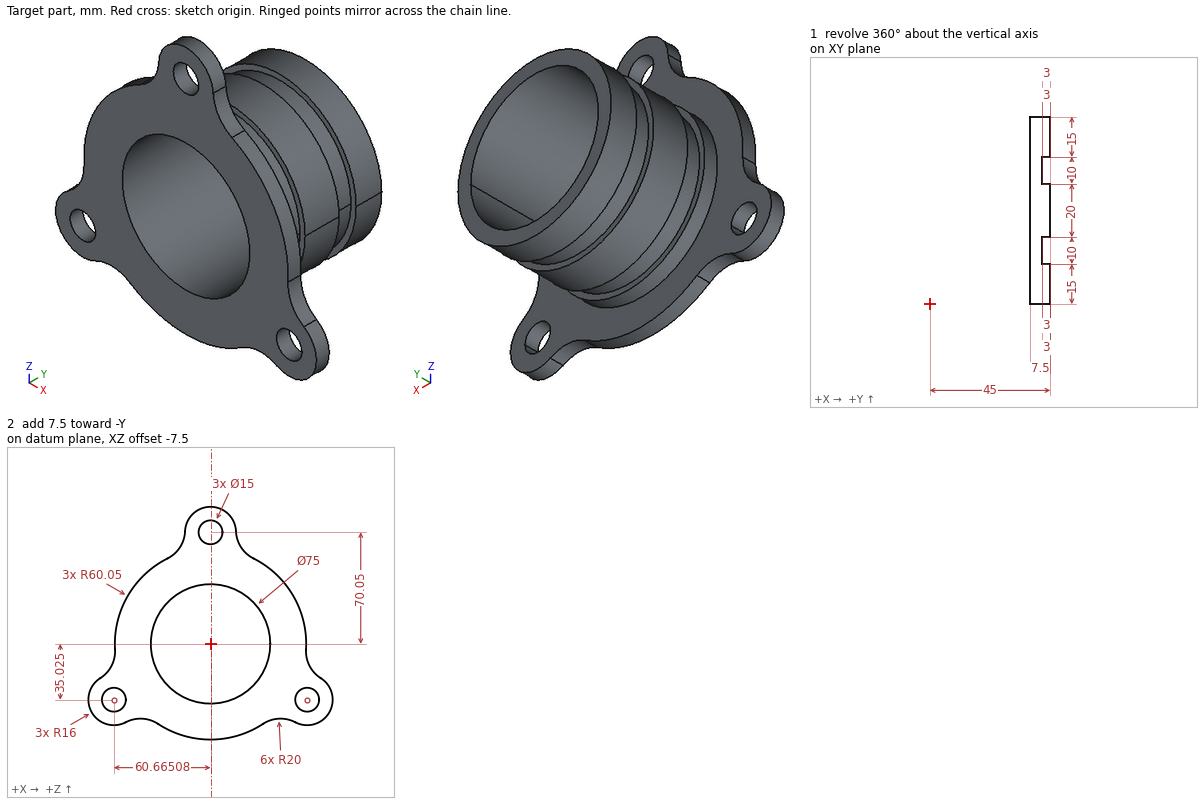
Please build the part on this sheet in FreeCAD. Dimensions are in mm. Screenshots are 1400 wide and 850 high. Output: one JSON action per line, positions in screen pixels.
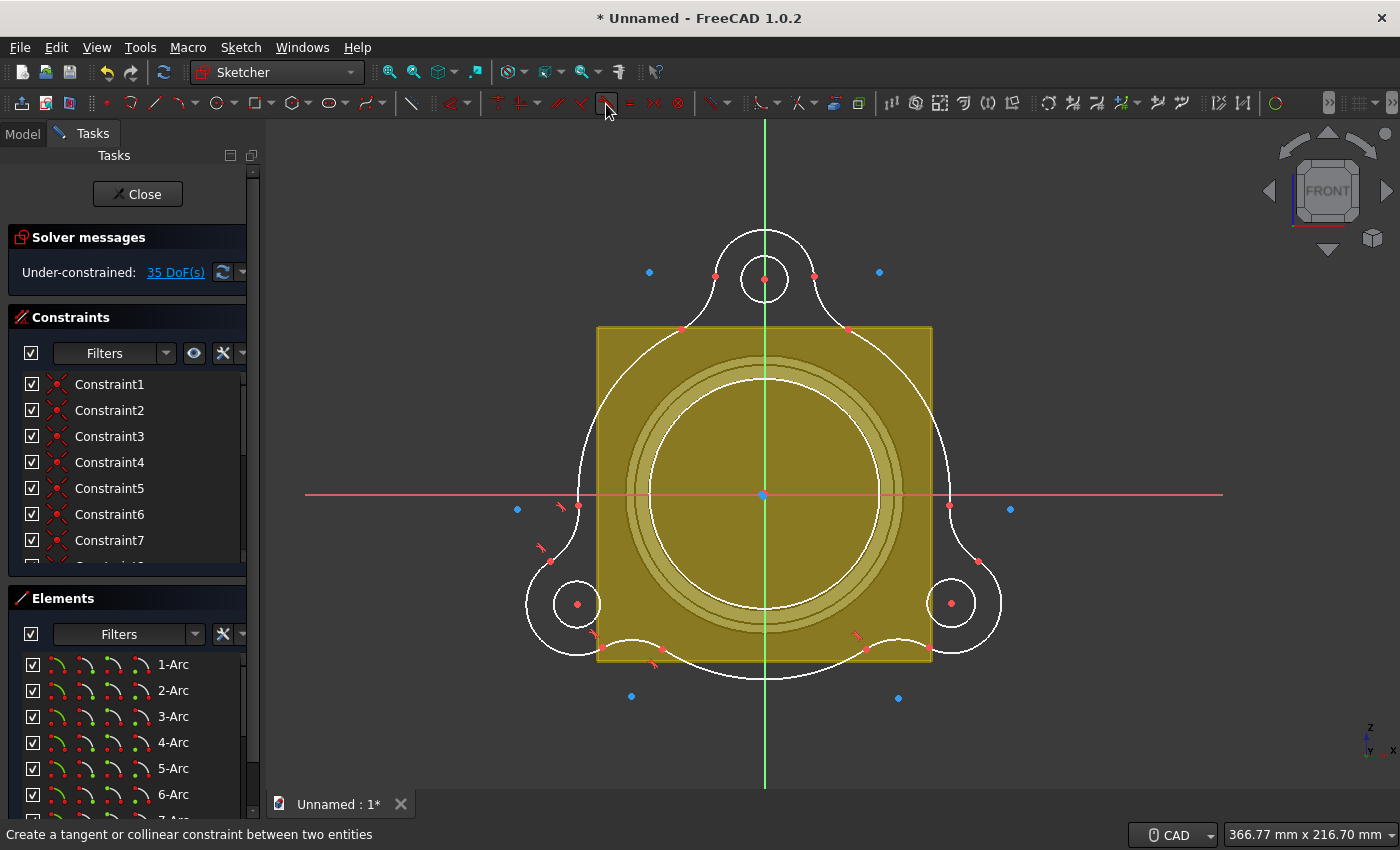
{"action": "left_click", "coordinate": [911, 641]}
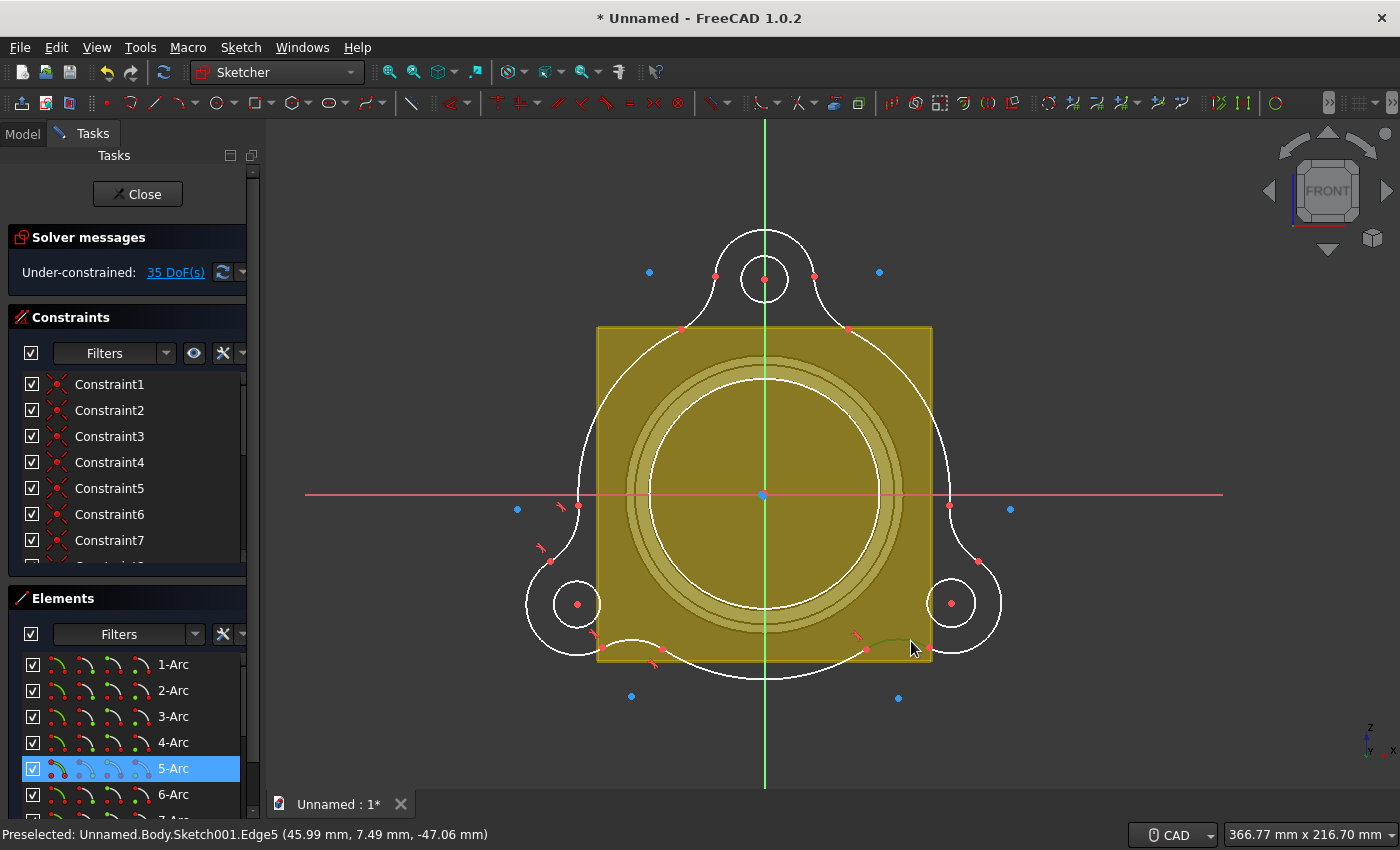
{"action": "left_click", "coordinate": [973, 648]}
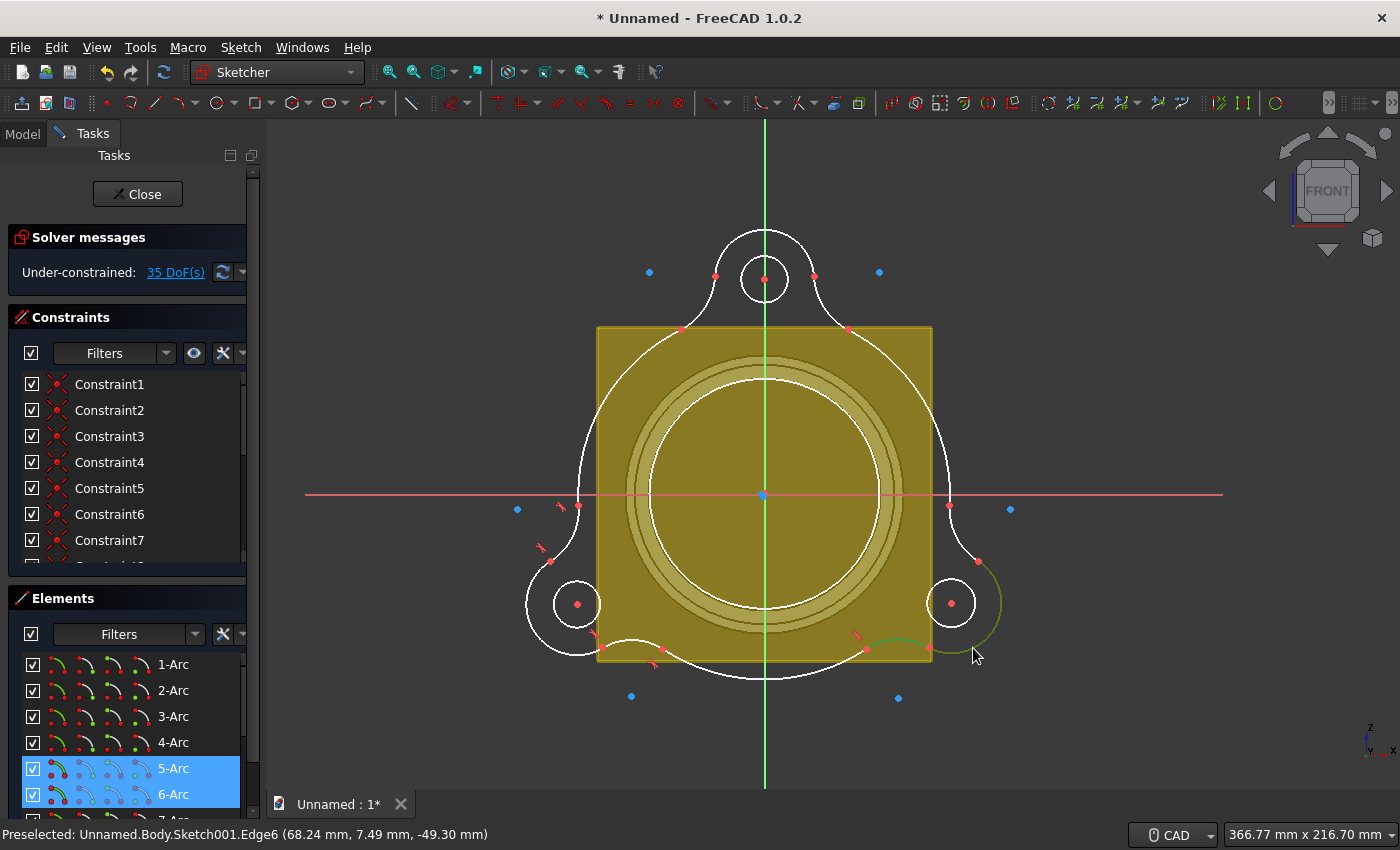
{"action": "left_click", "coordinate": [606, 104]}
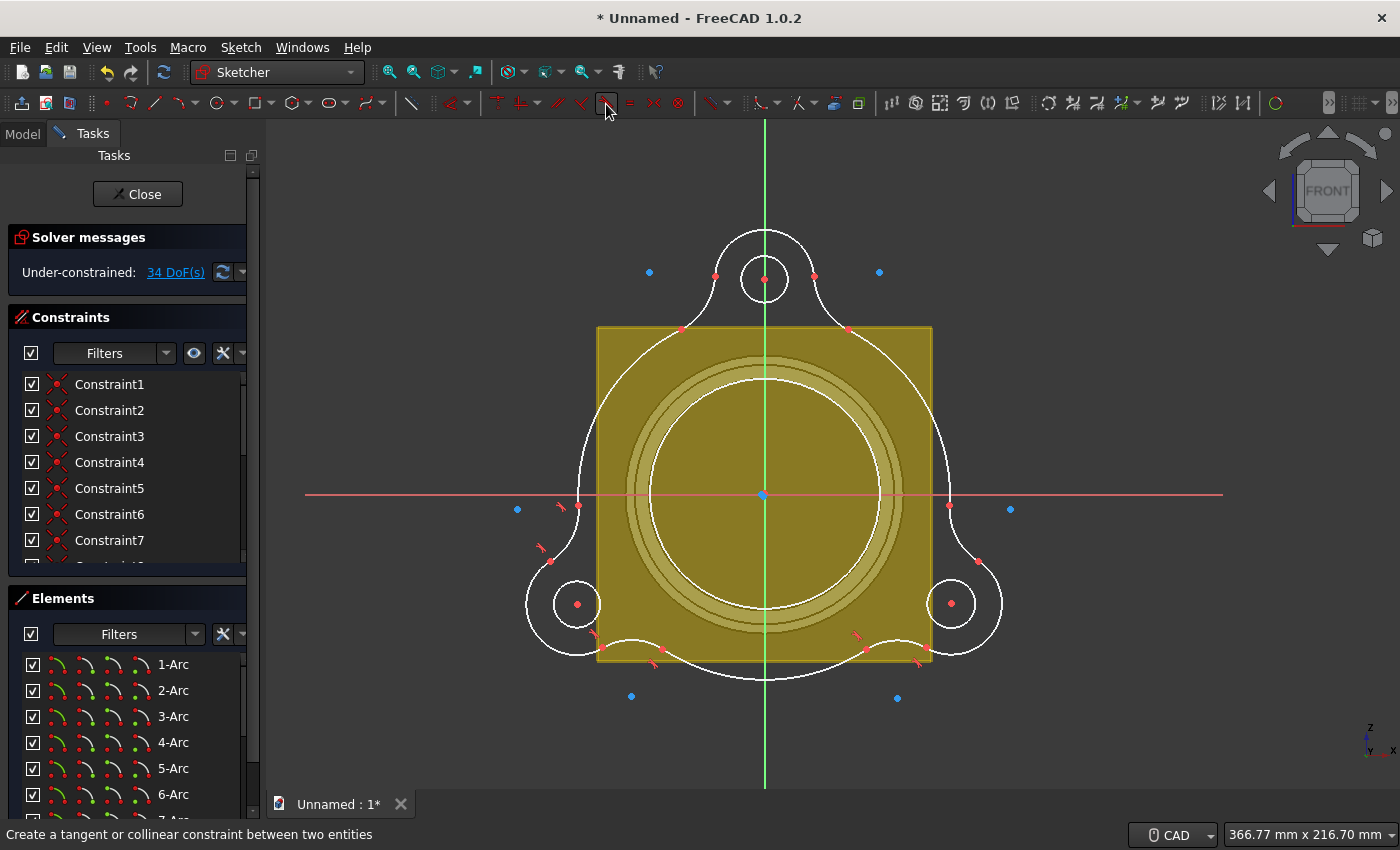
{"action": "left_click", "coordinate": [971, 650]}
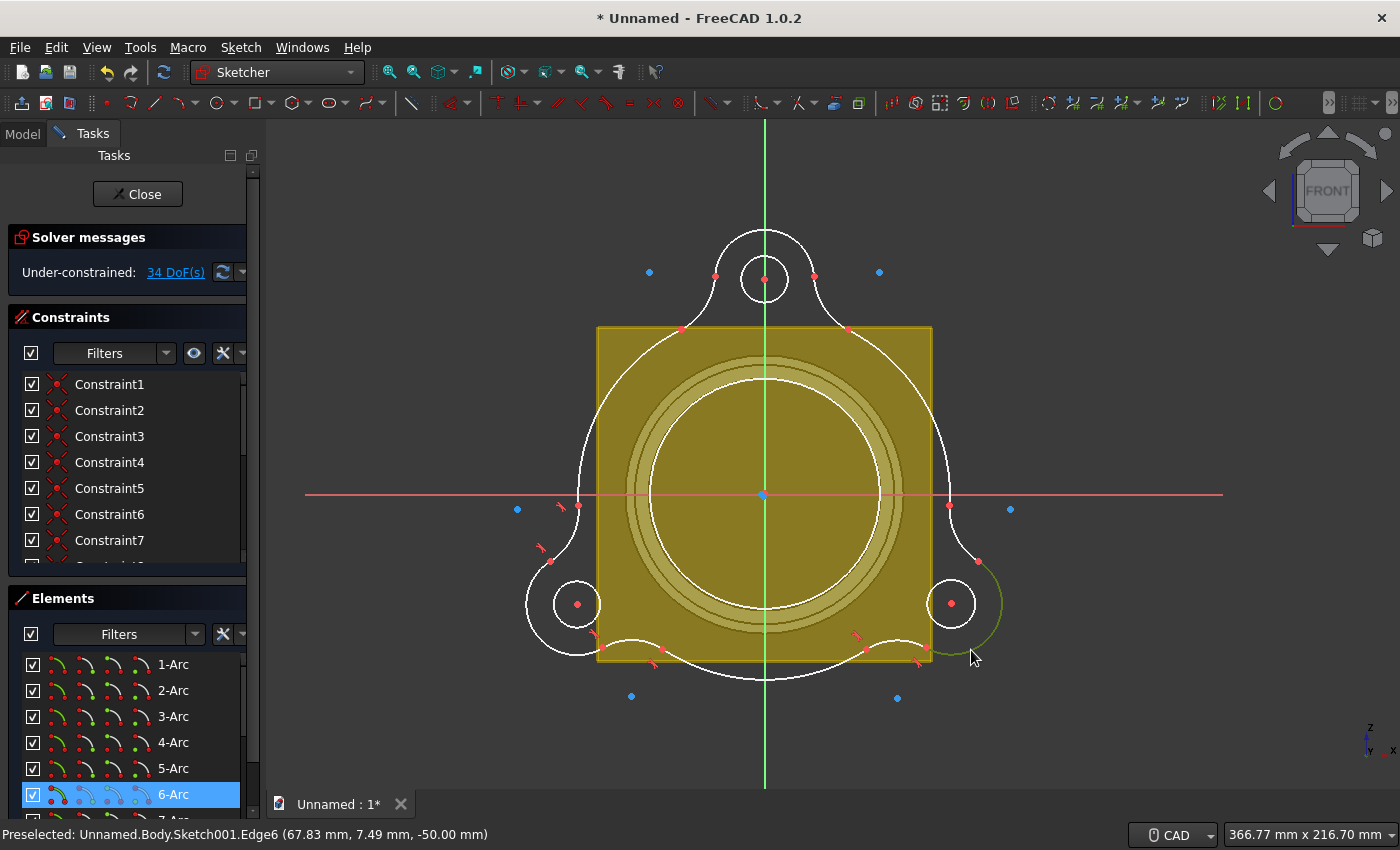
{"action": "left_click", "coordinate": [952, 525]}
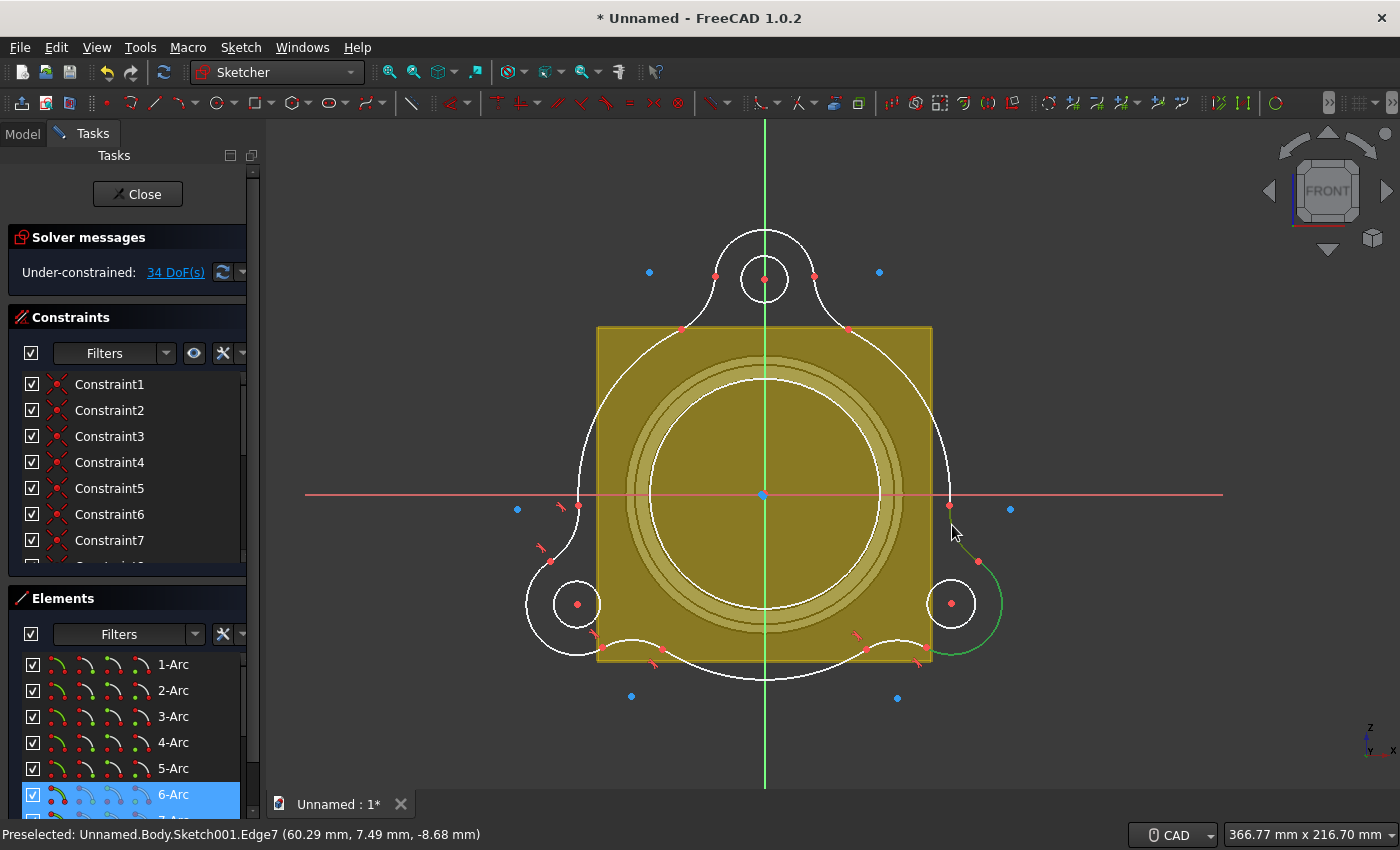
{"action": "left_click", "coordinate": [606, 104]}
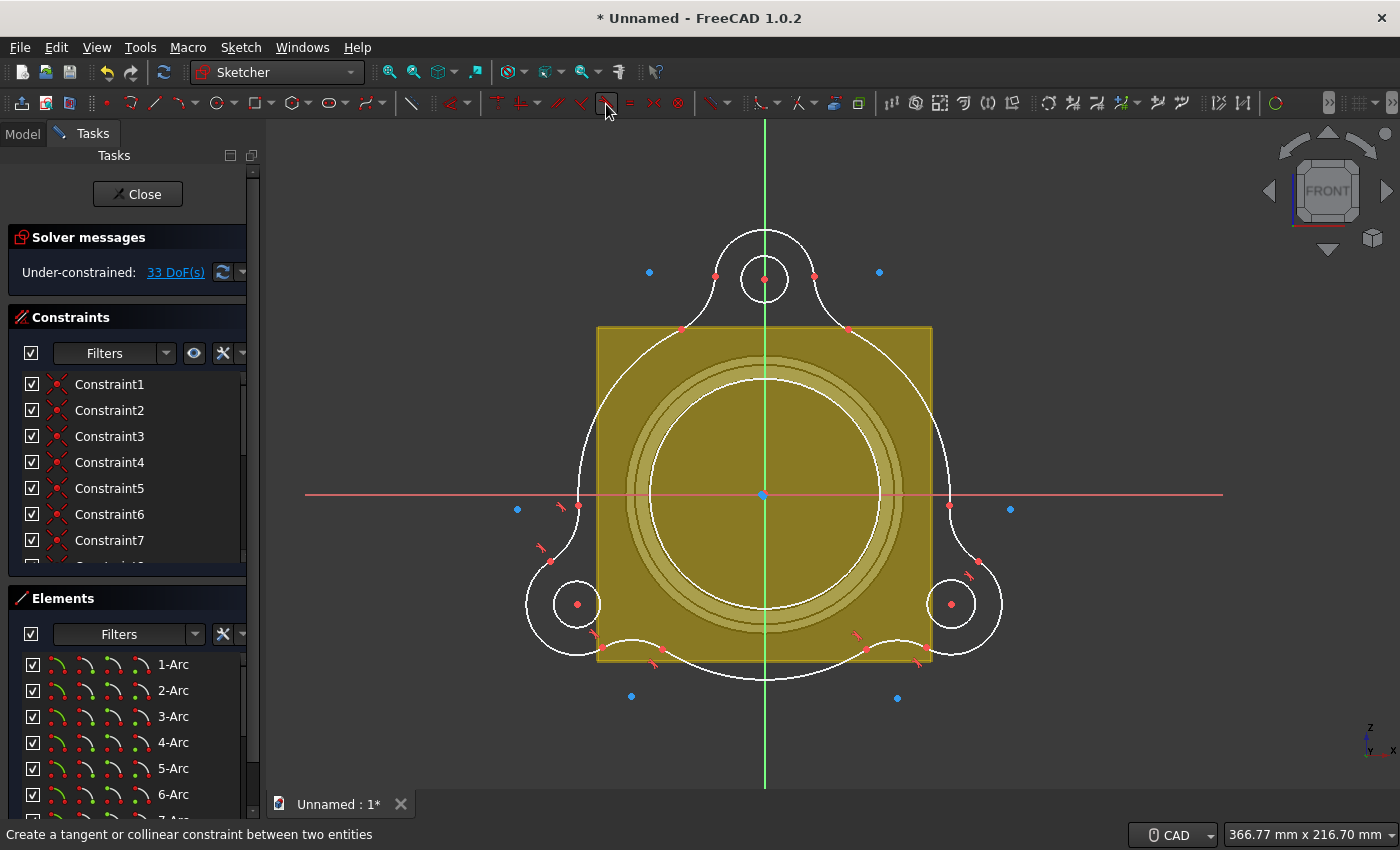
{"action": "left_click", "coordinate": [952, 525]}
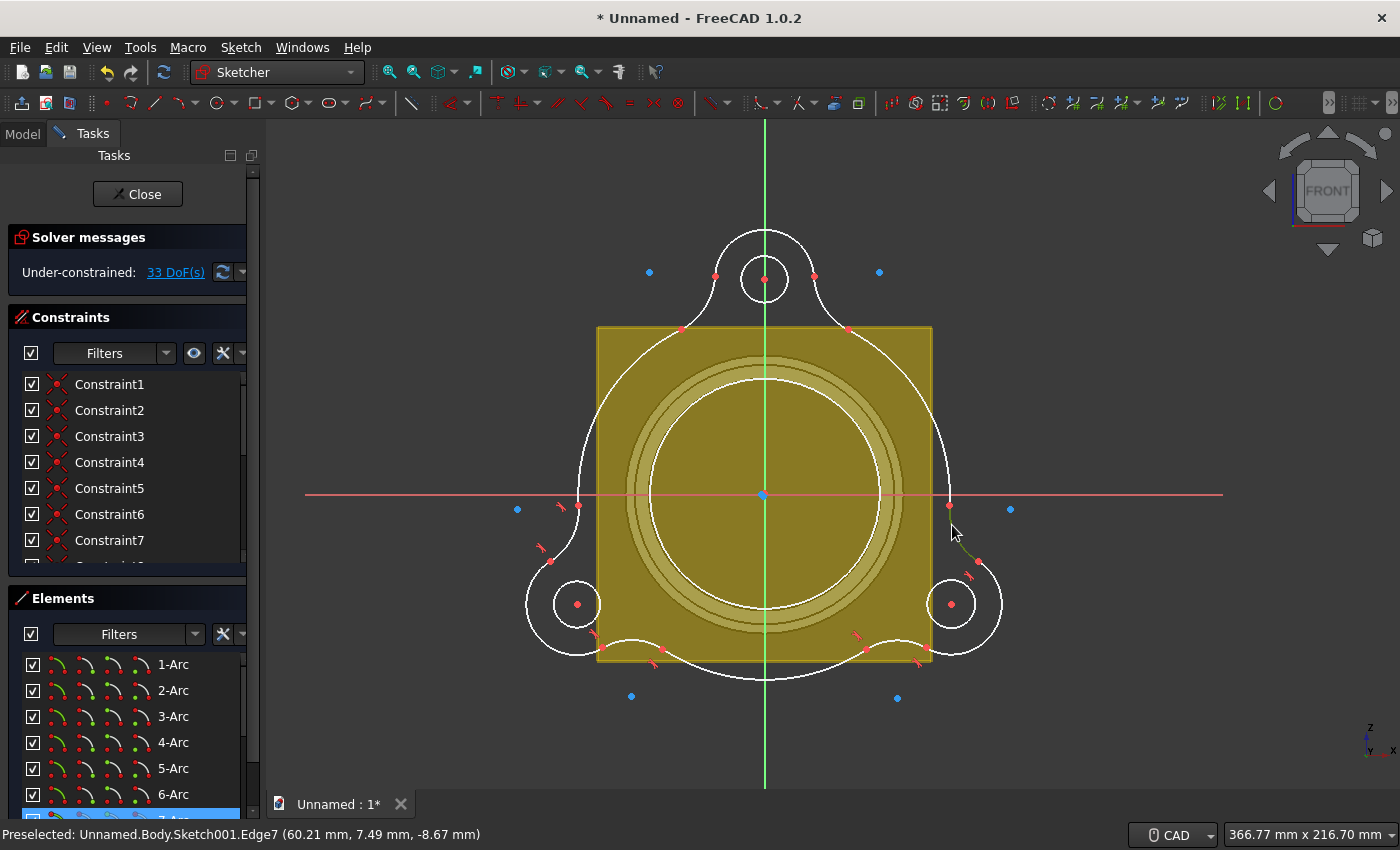
{"action": "left_click", "coordinate": [942, 442]}